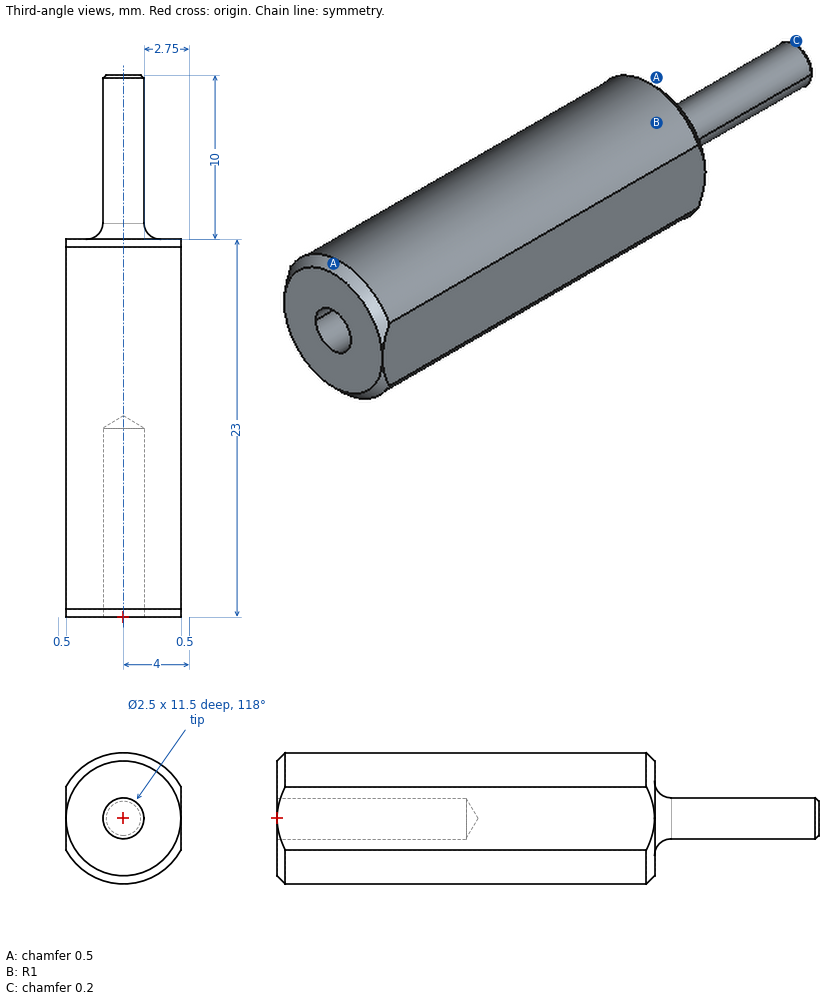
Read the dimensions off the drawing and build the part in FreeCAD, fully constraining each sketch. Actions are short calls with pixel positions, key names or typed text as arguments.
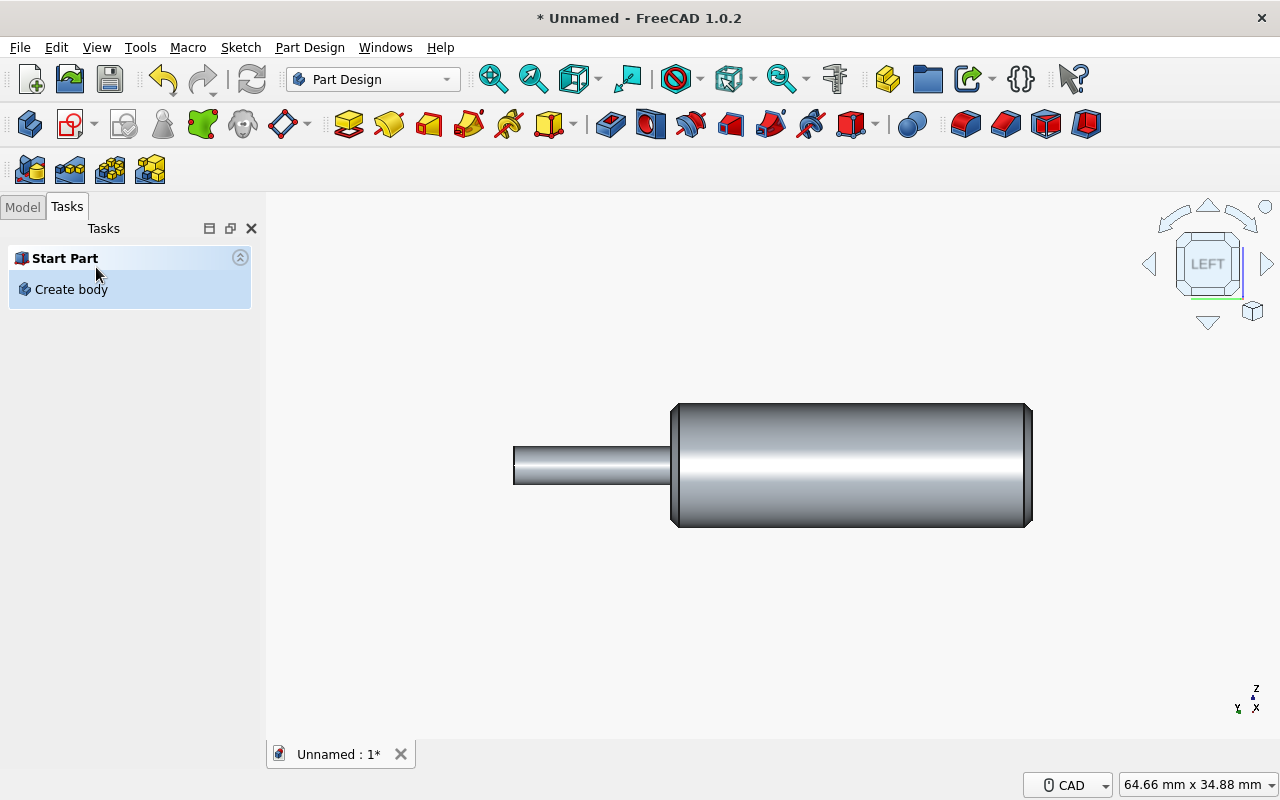
key(v)
key(3)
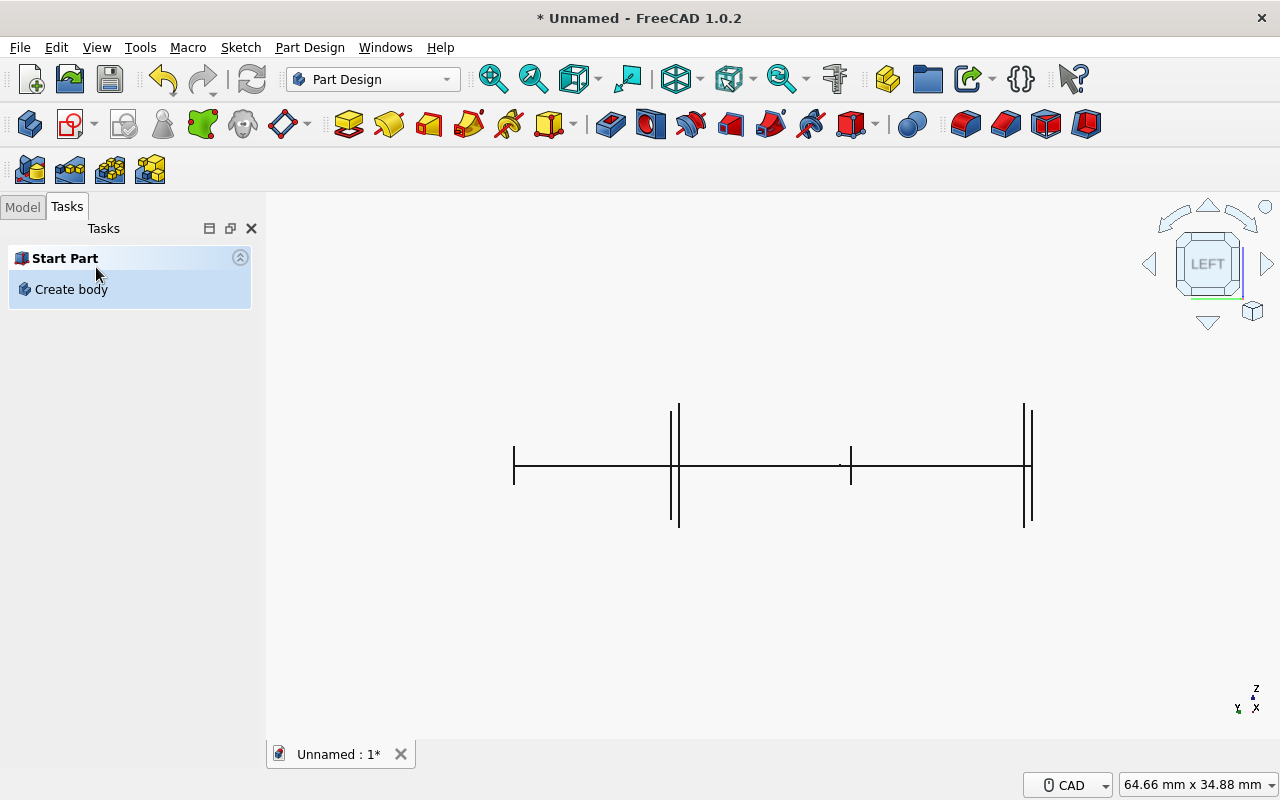
key(0)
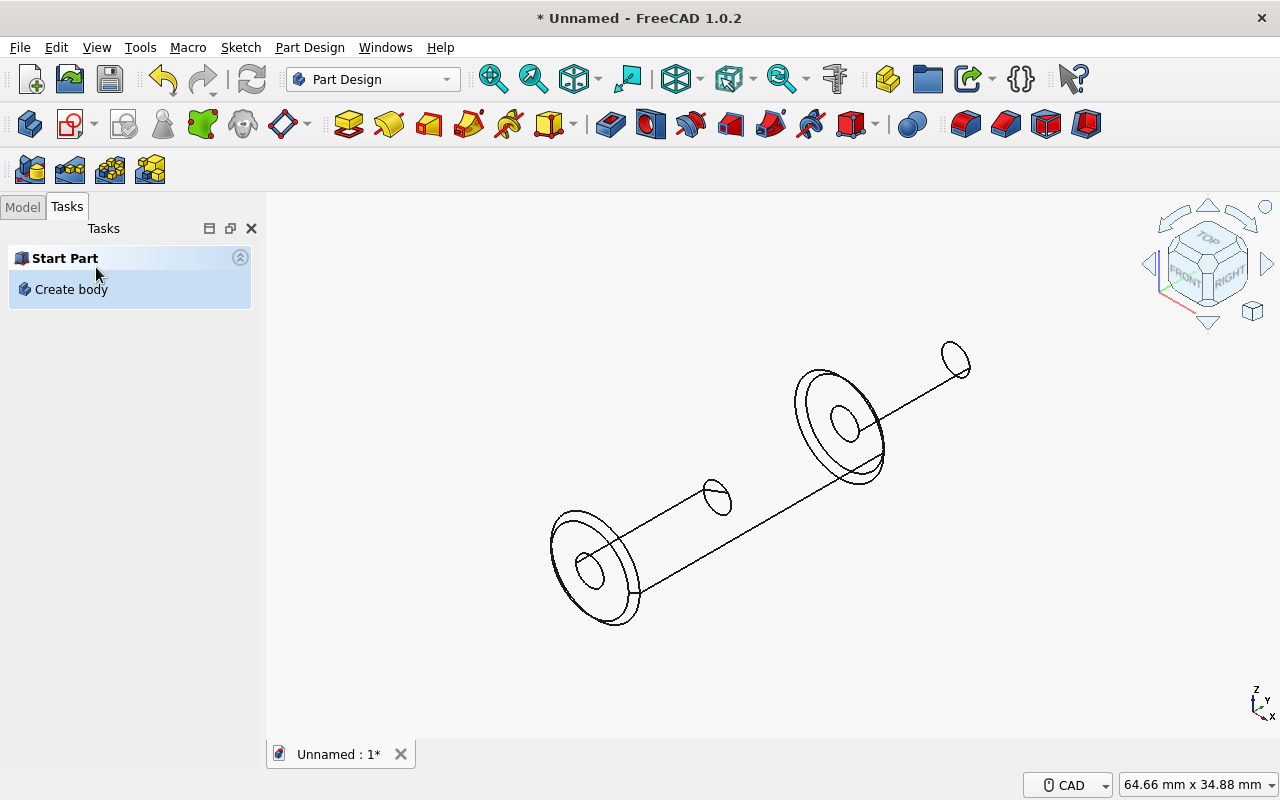
click(831, 415)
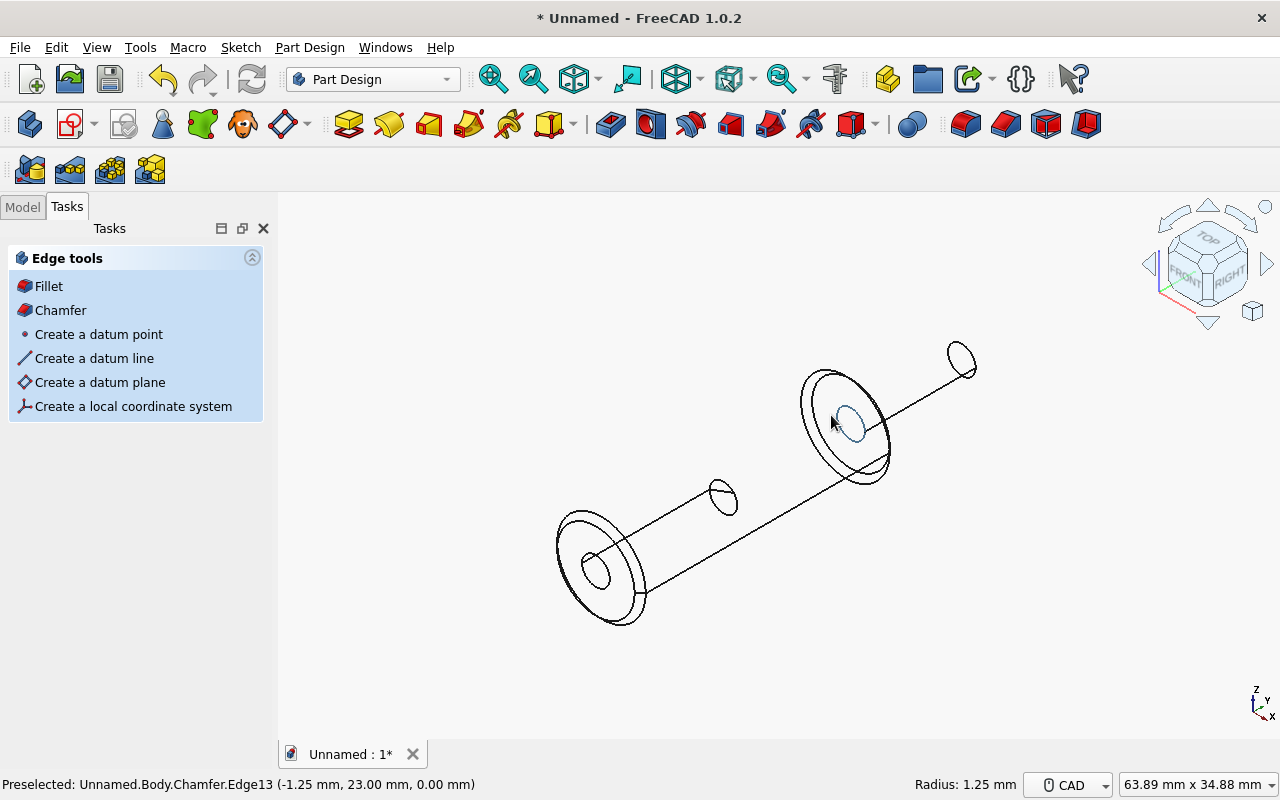
key(v)
key(1)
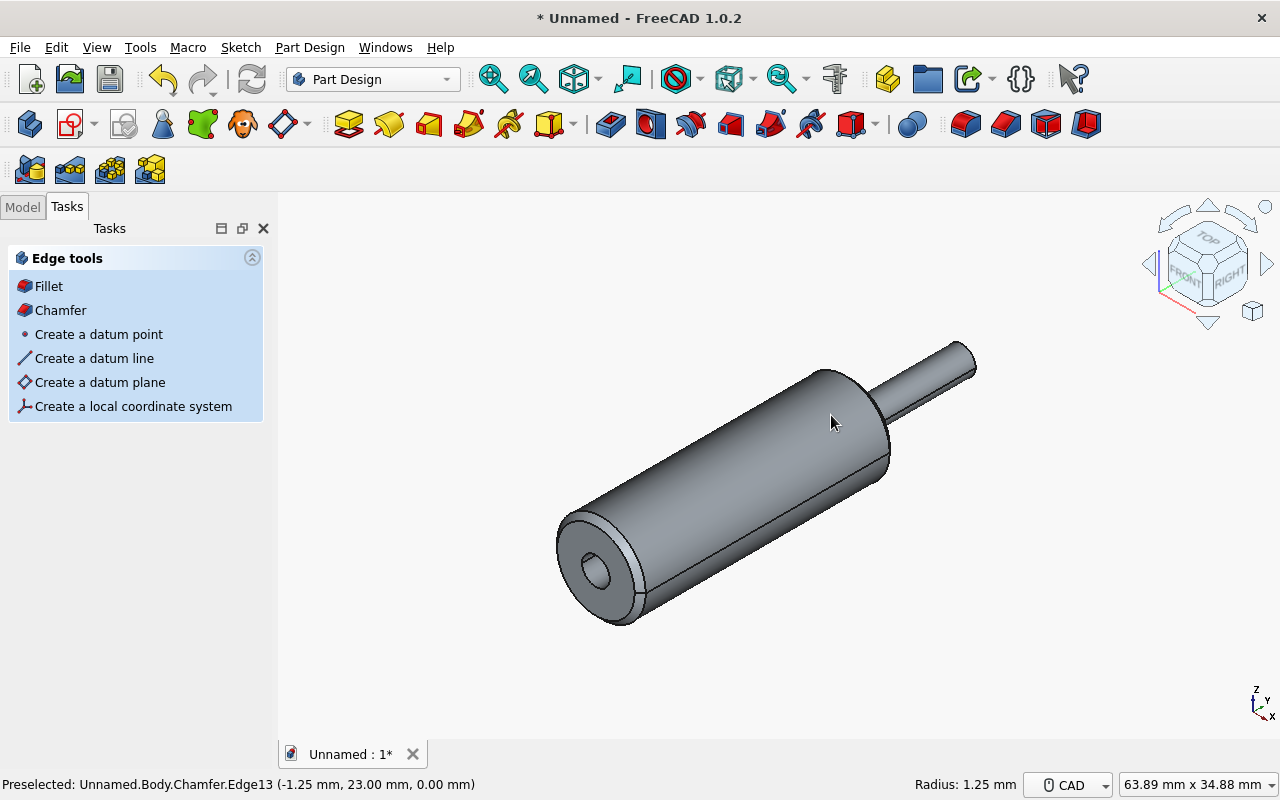
click(966, 124)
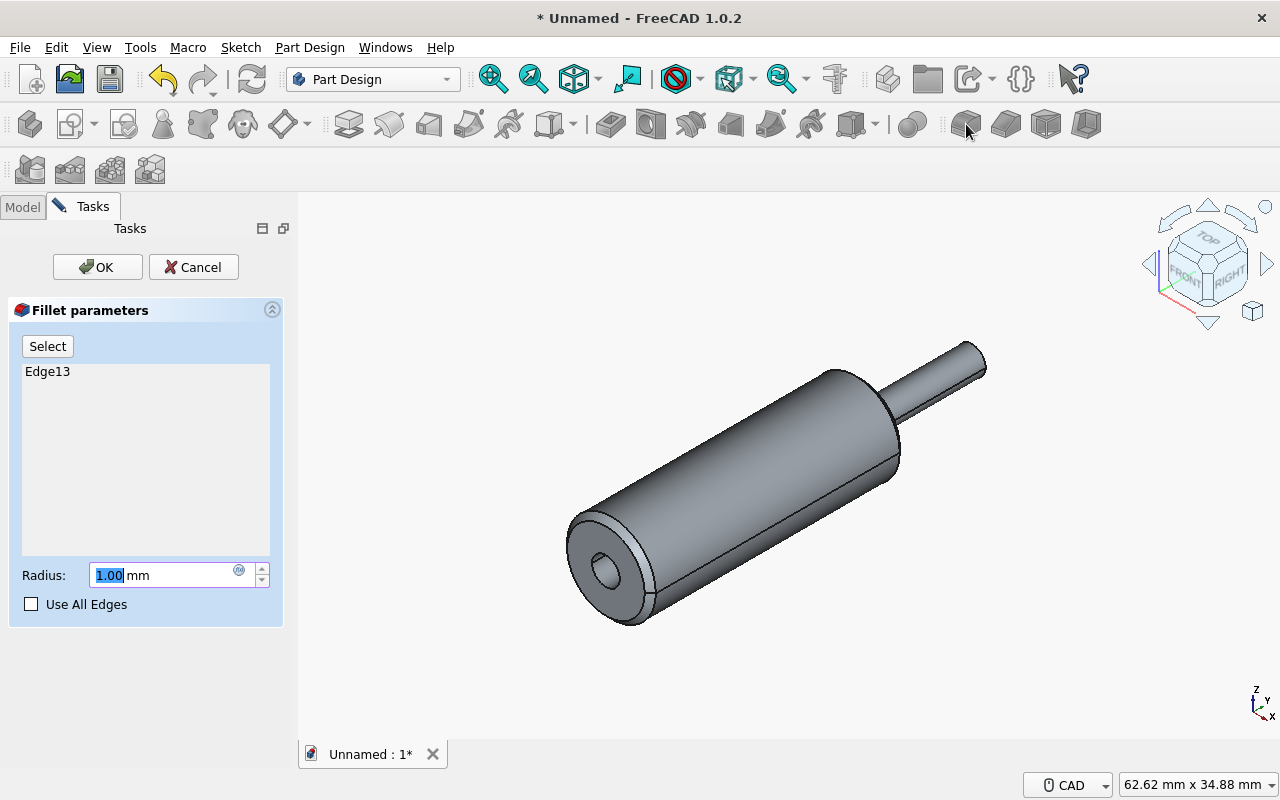
text(1)
key(Tab)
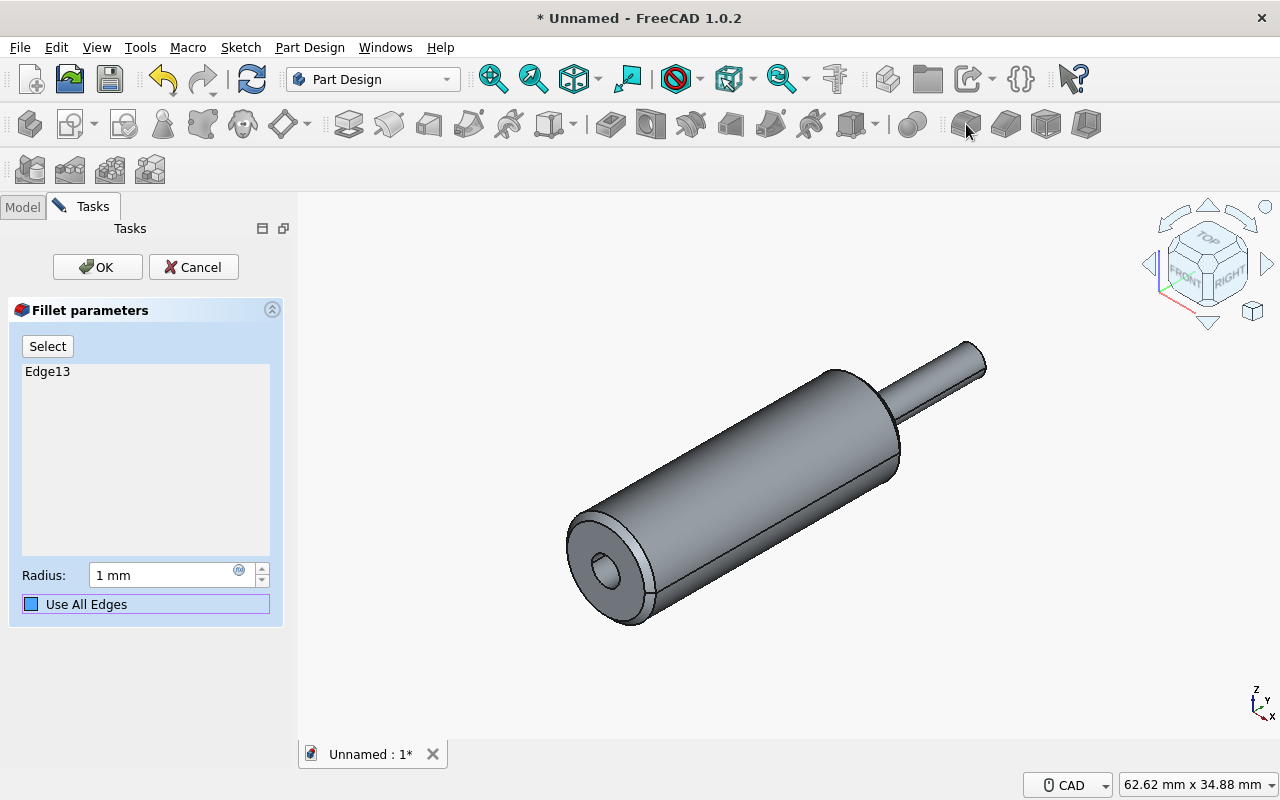
click(98, 267)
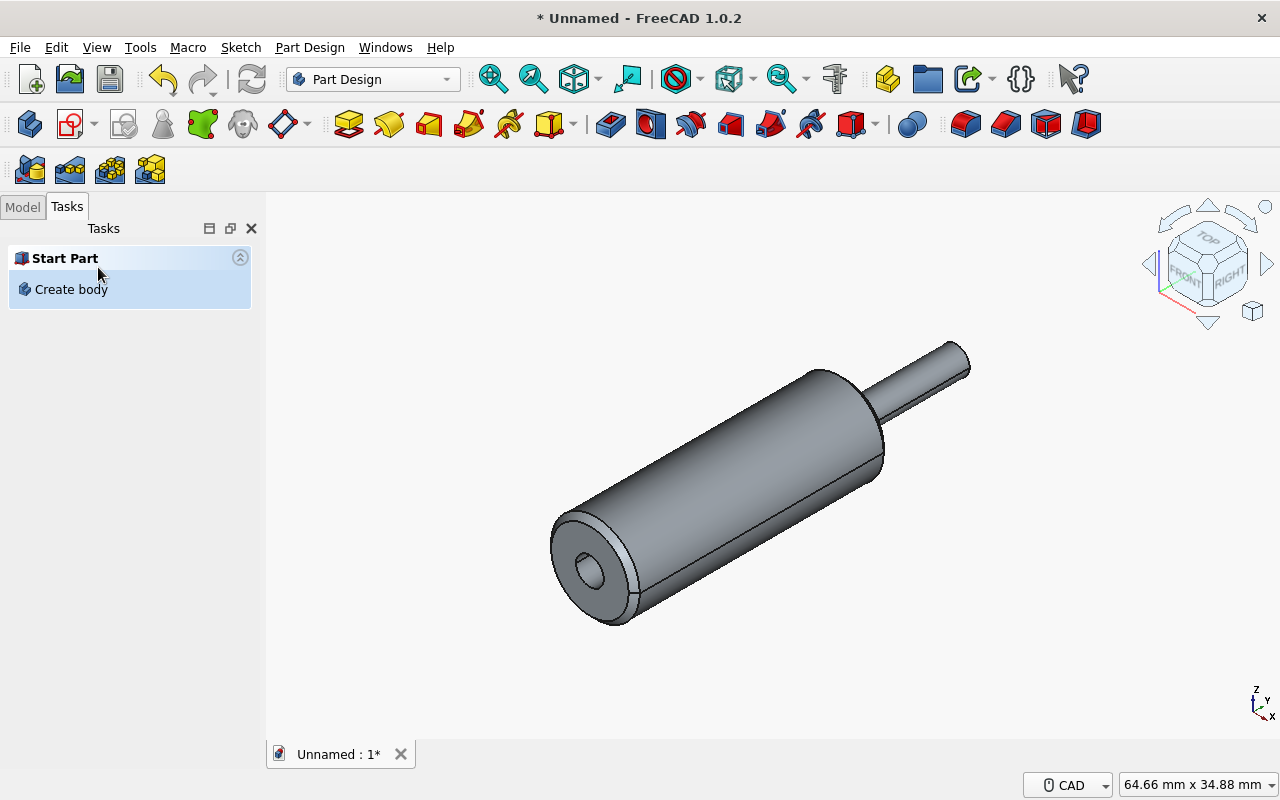
click(70, 124)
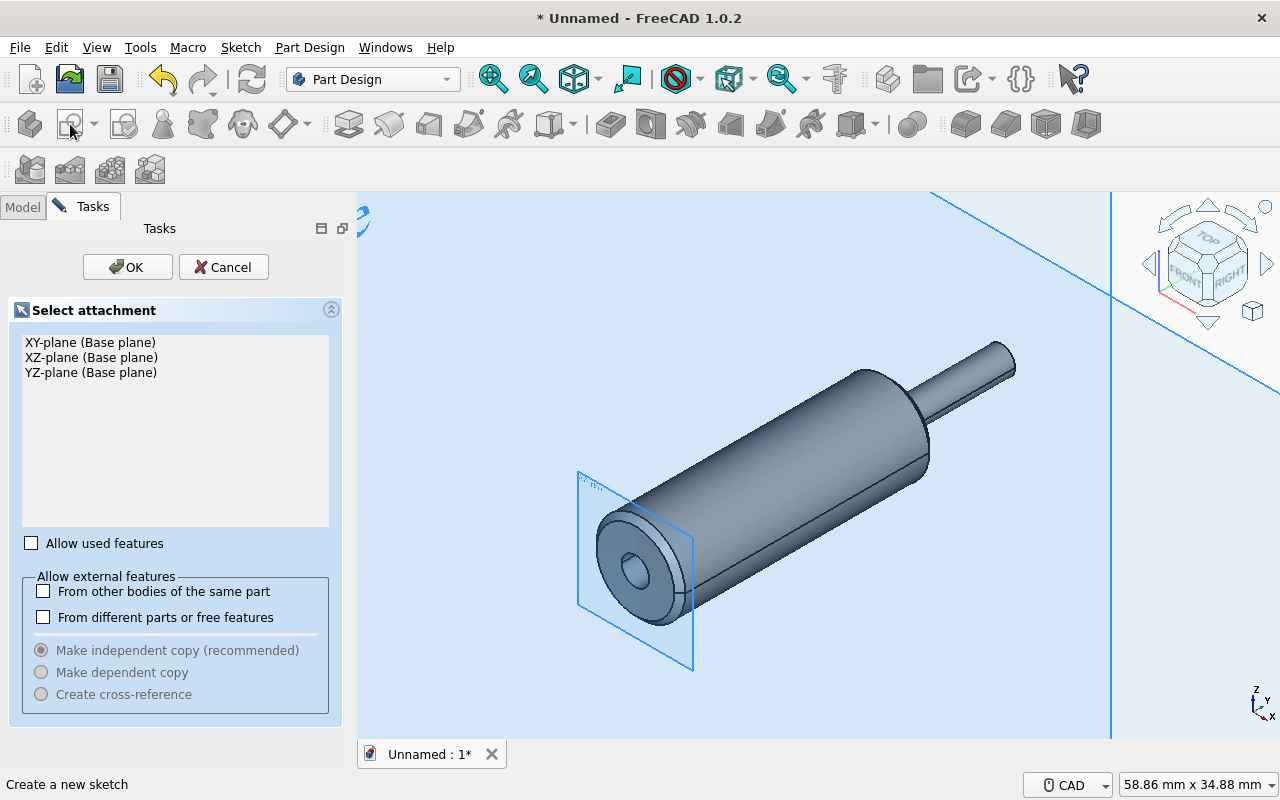
click(82, 342)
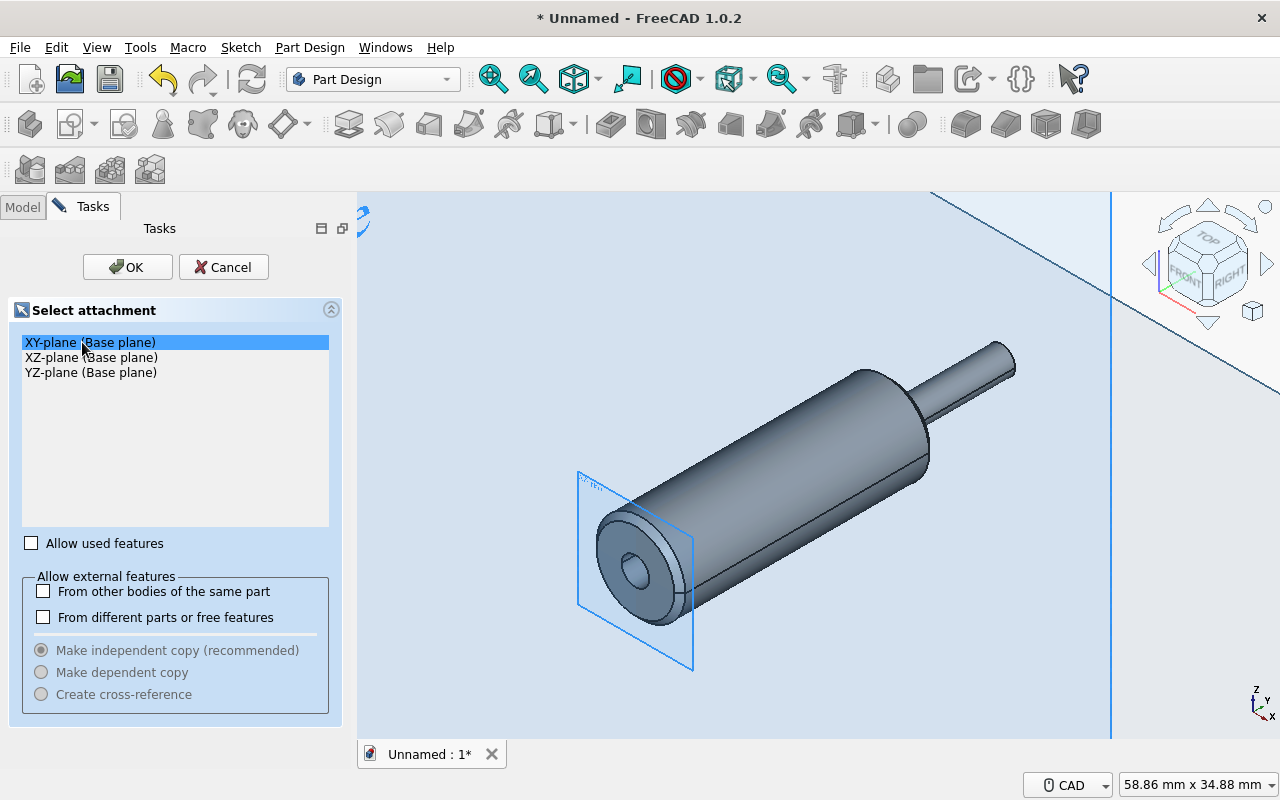
click(128, 267)